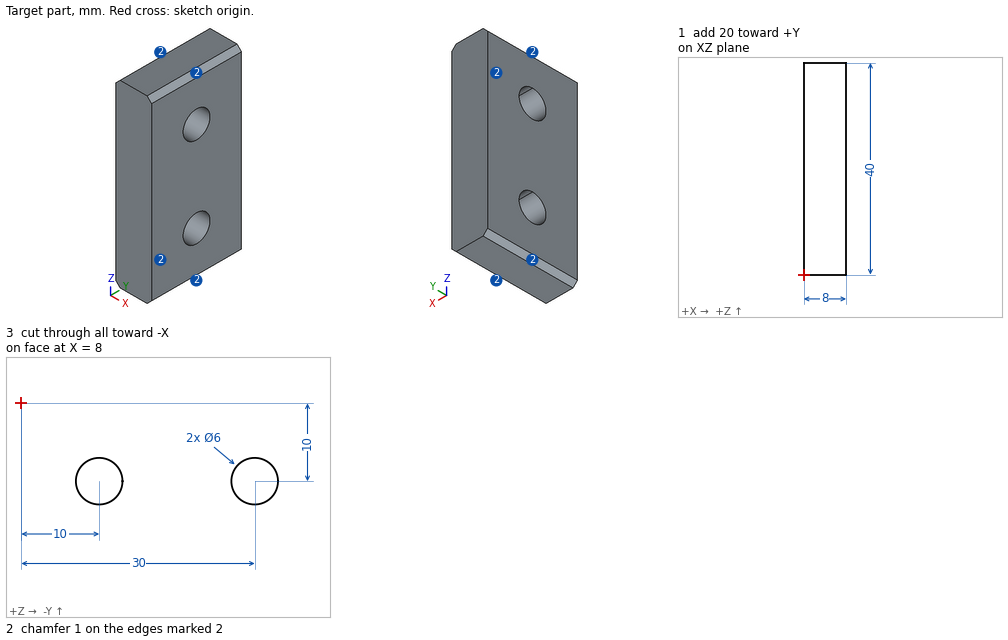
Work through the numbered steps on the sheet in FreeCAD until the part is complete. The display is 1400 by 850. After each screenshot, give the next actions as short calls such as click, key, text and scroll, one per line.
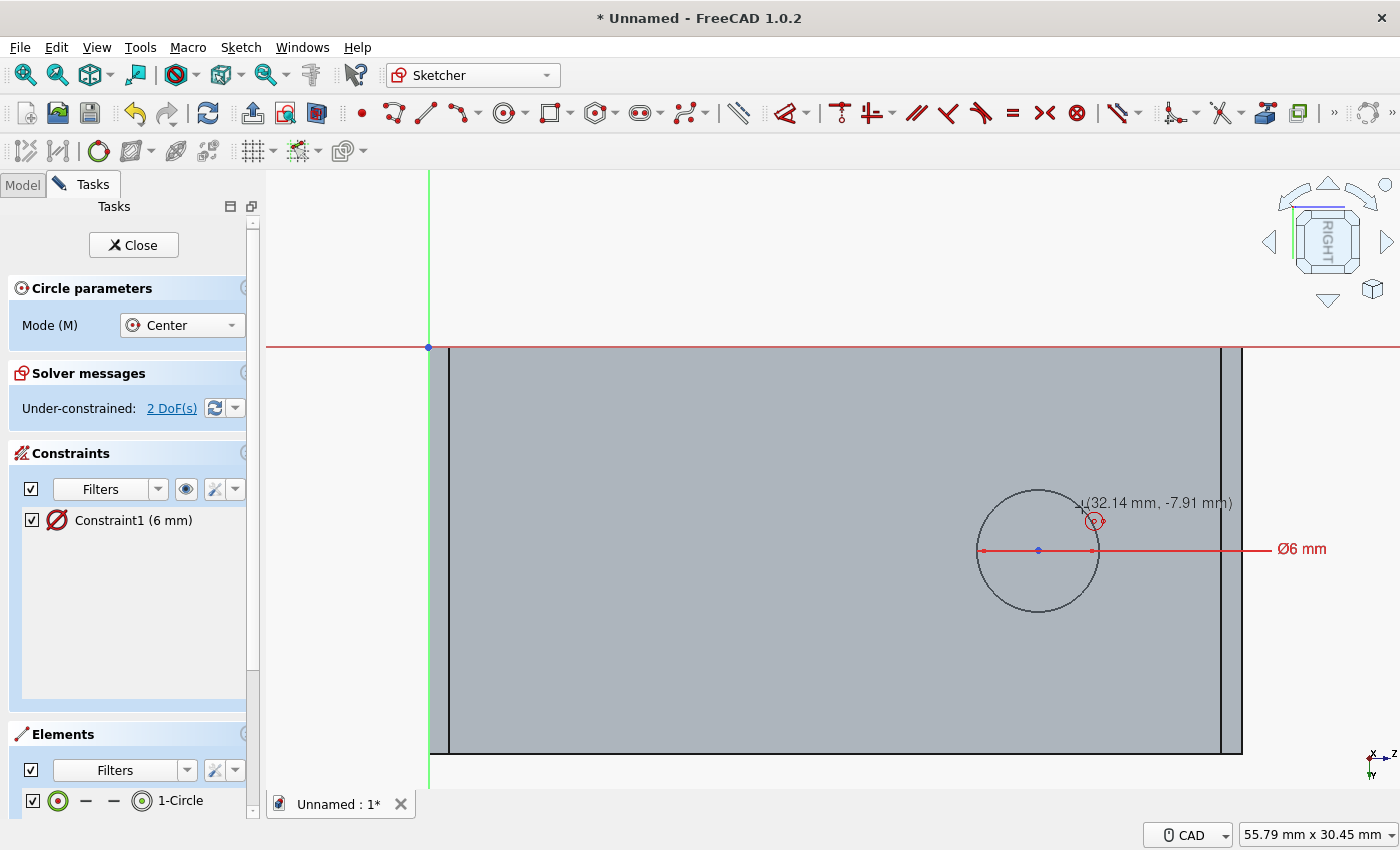
click(632, 550)
move(675, 507)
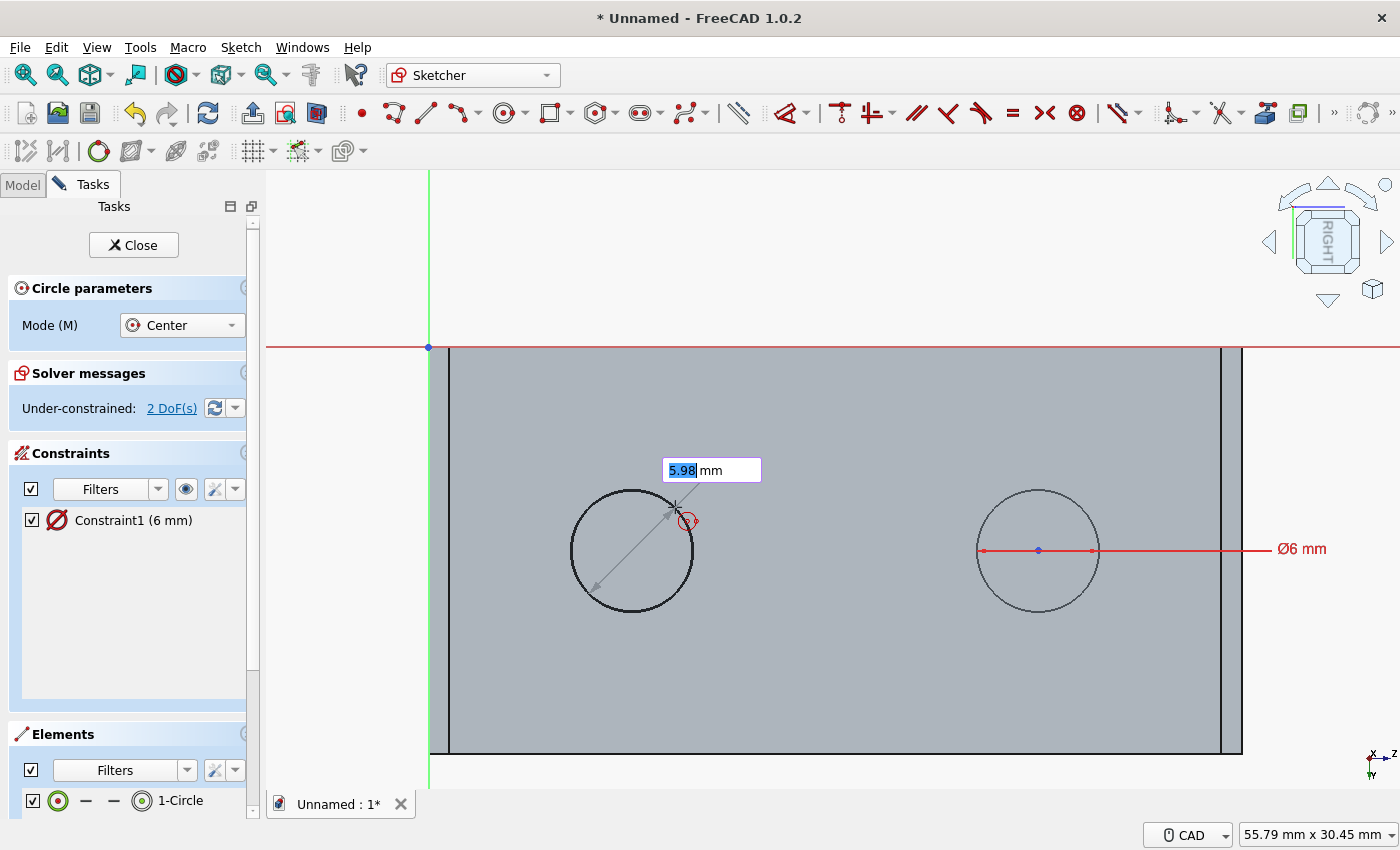
text(6)
key(Return)
key(Escape)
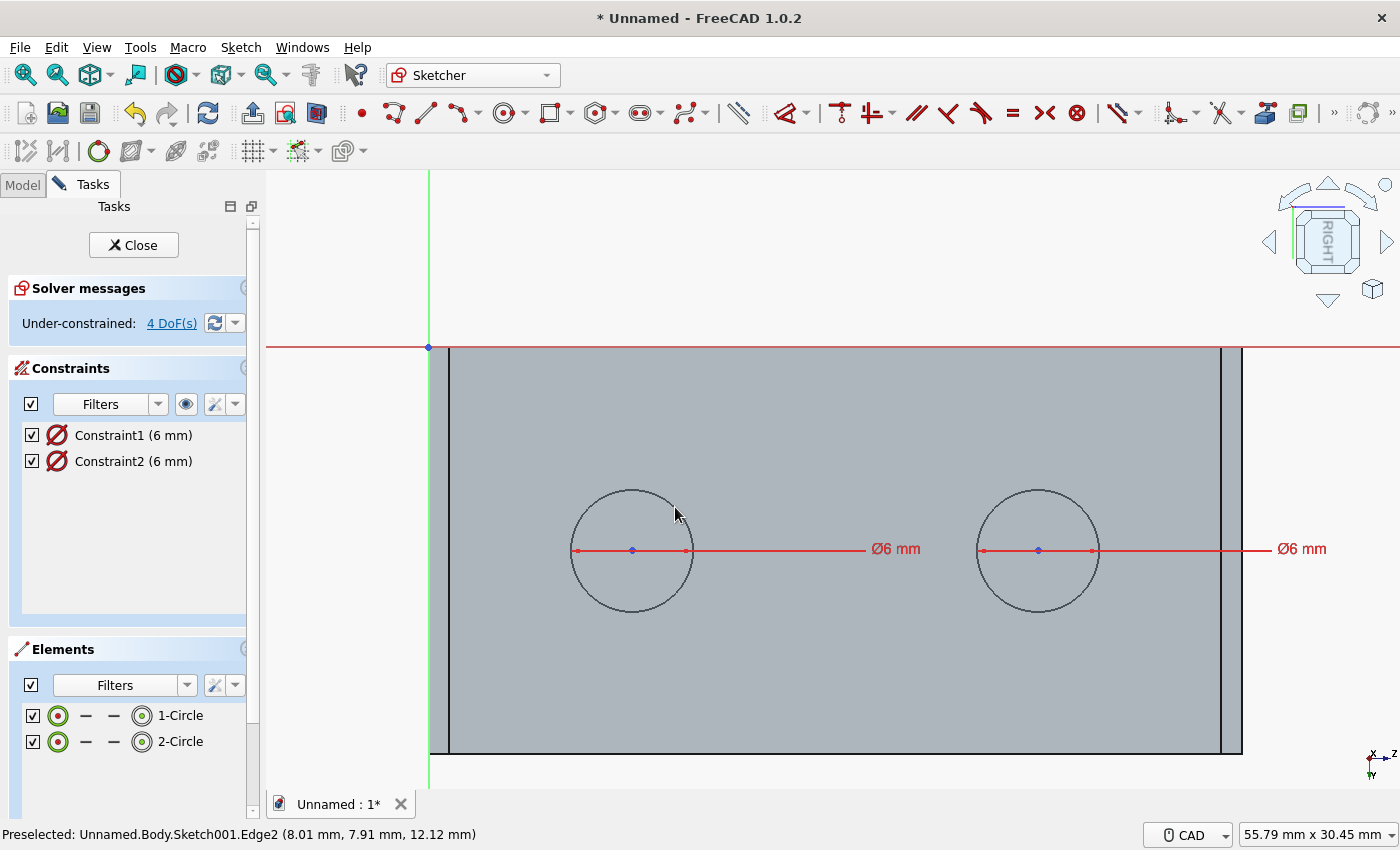
click(1038, 551)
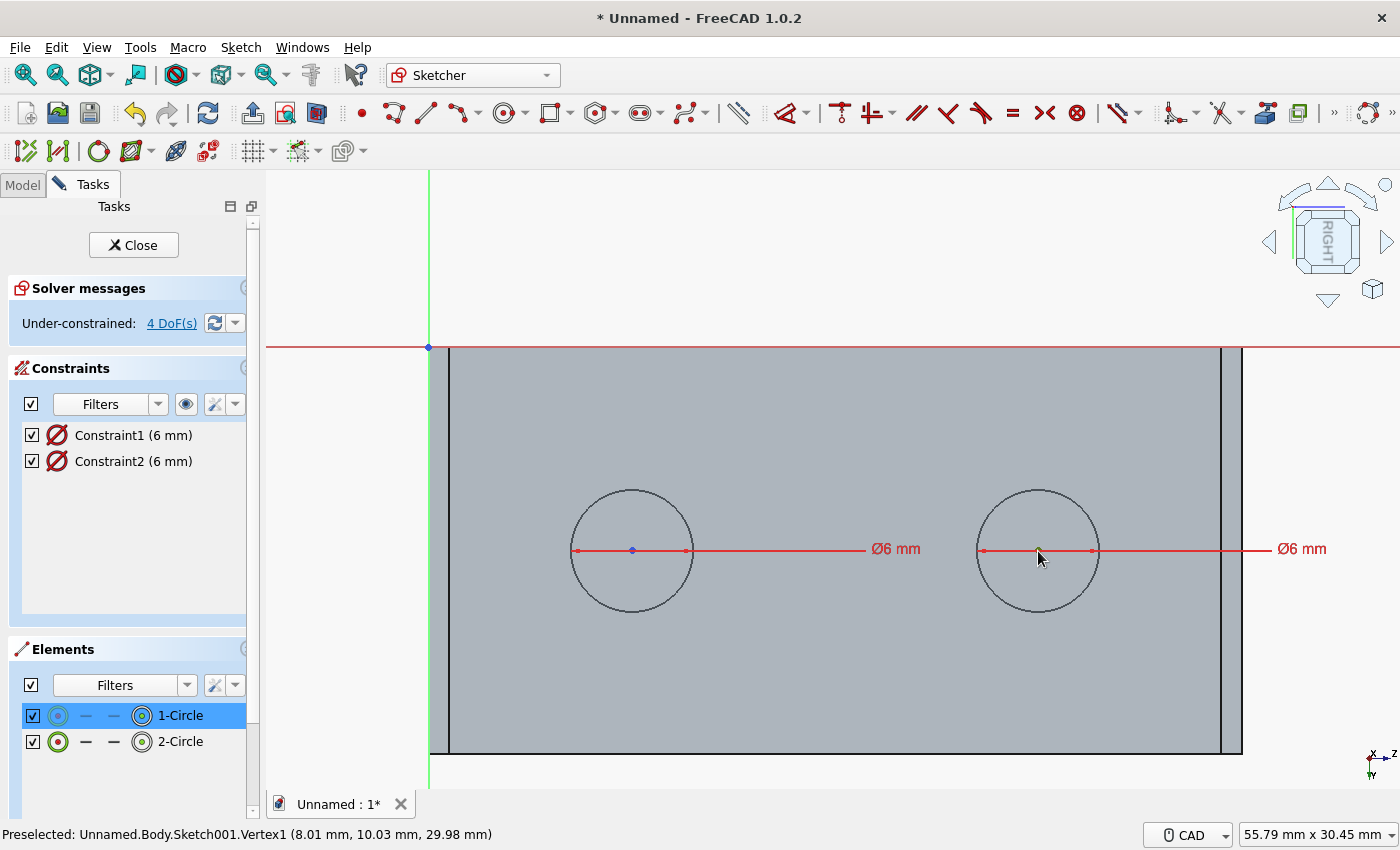
click(632, 551)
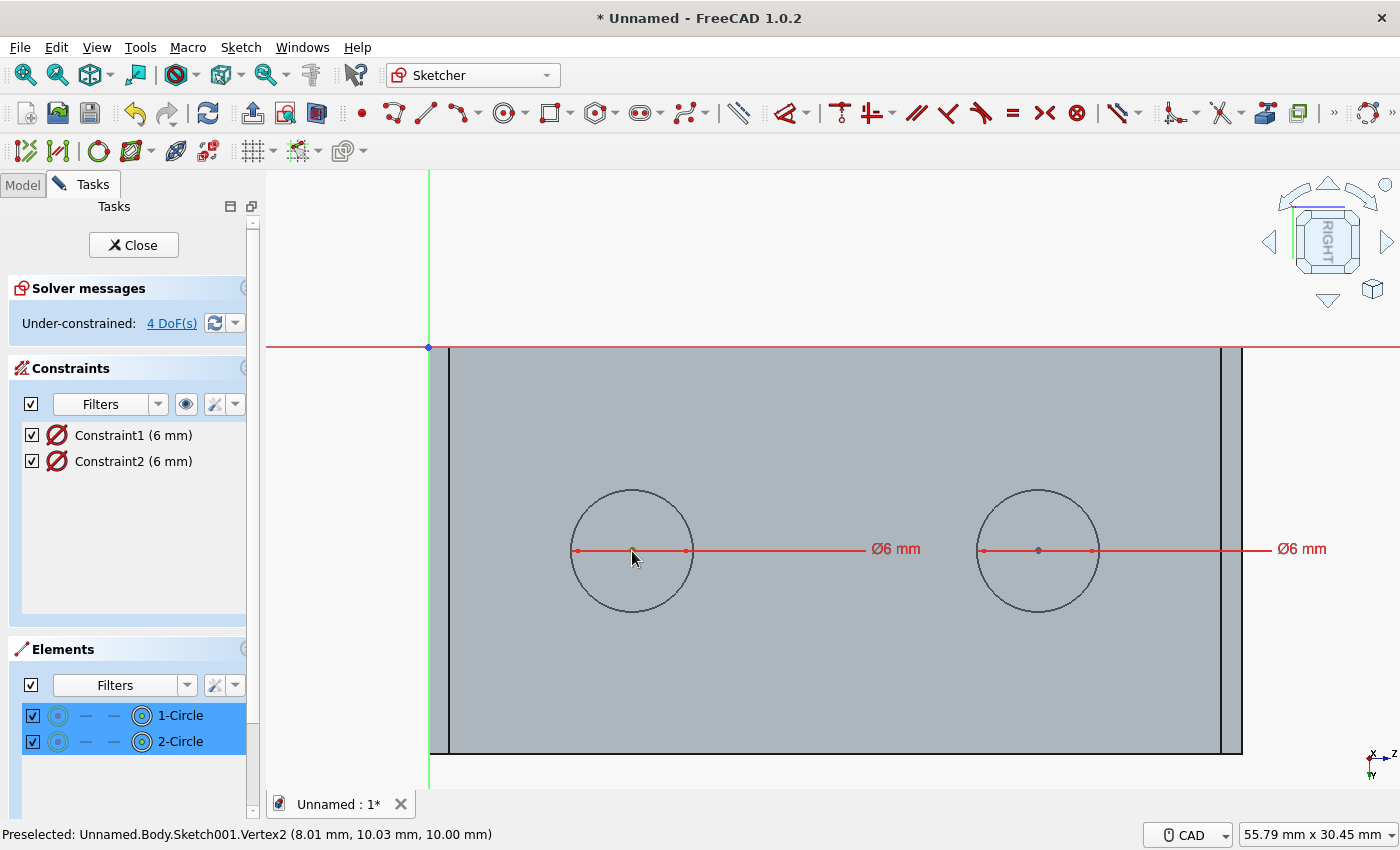
key(h)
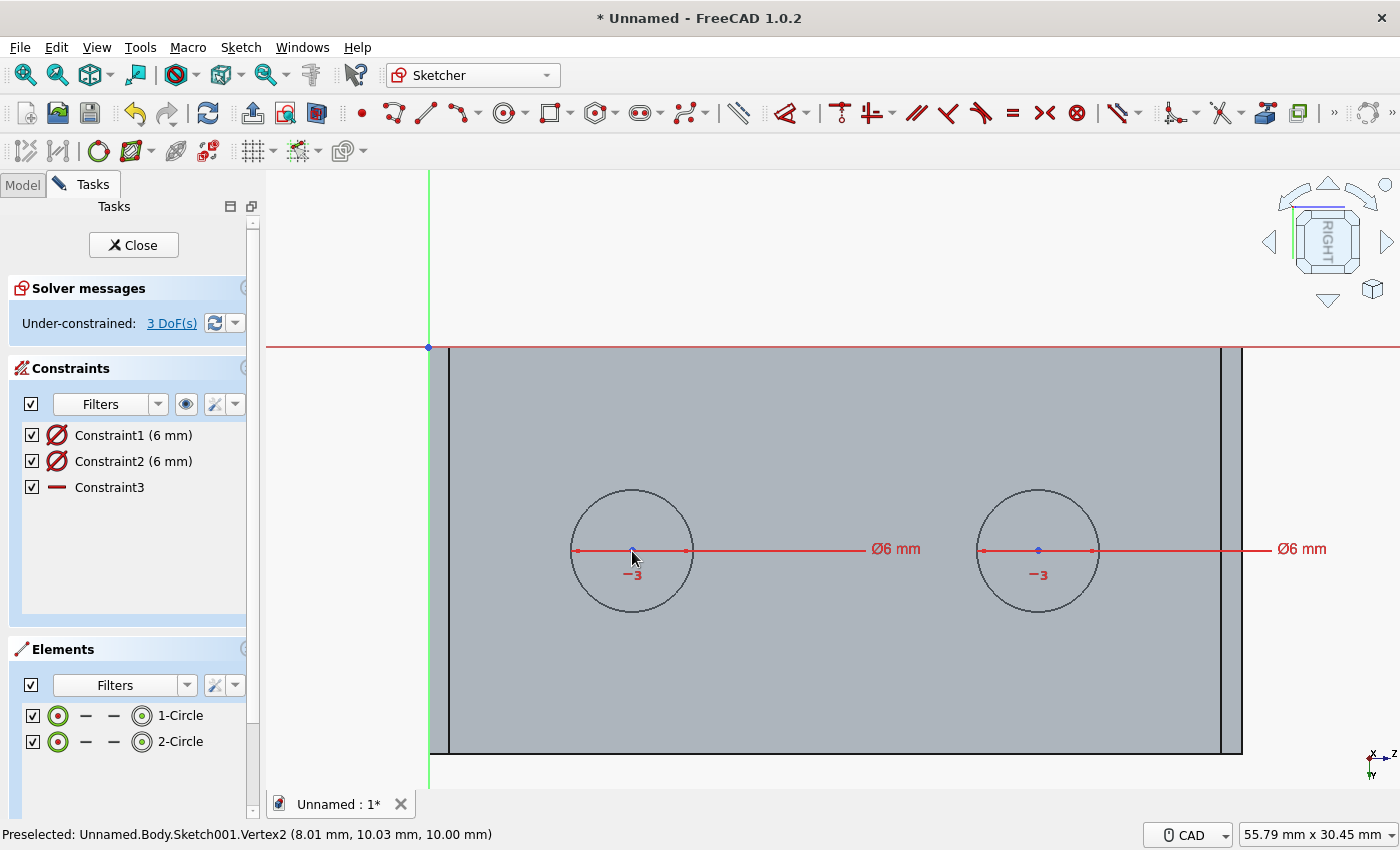
click(786, 114)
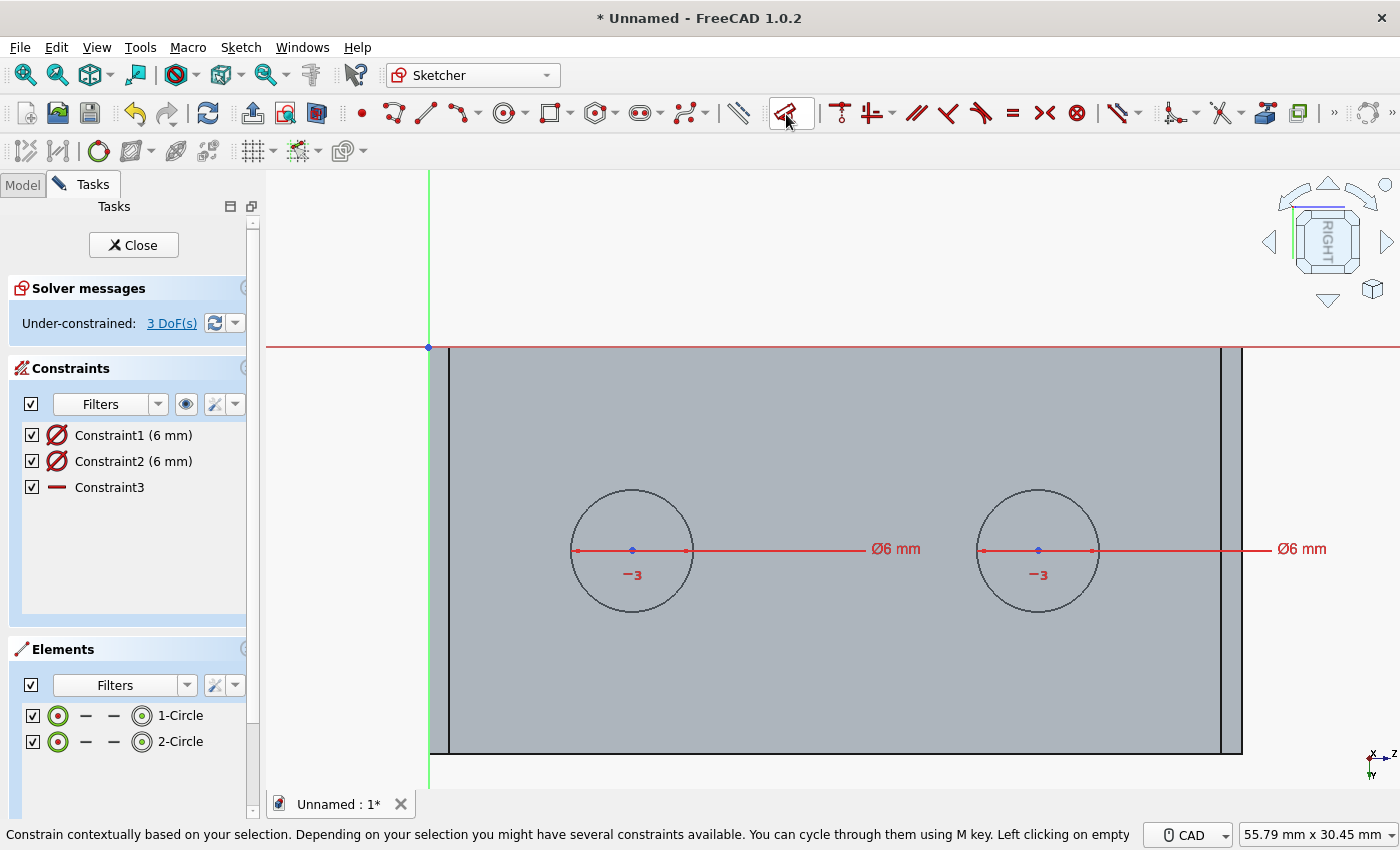
click(1038, 551)
click(733, 313)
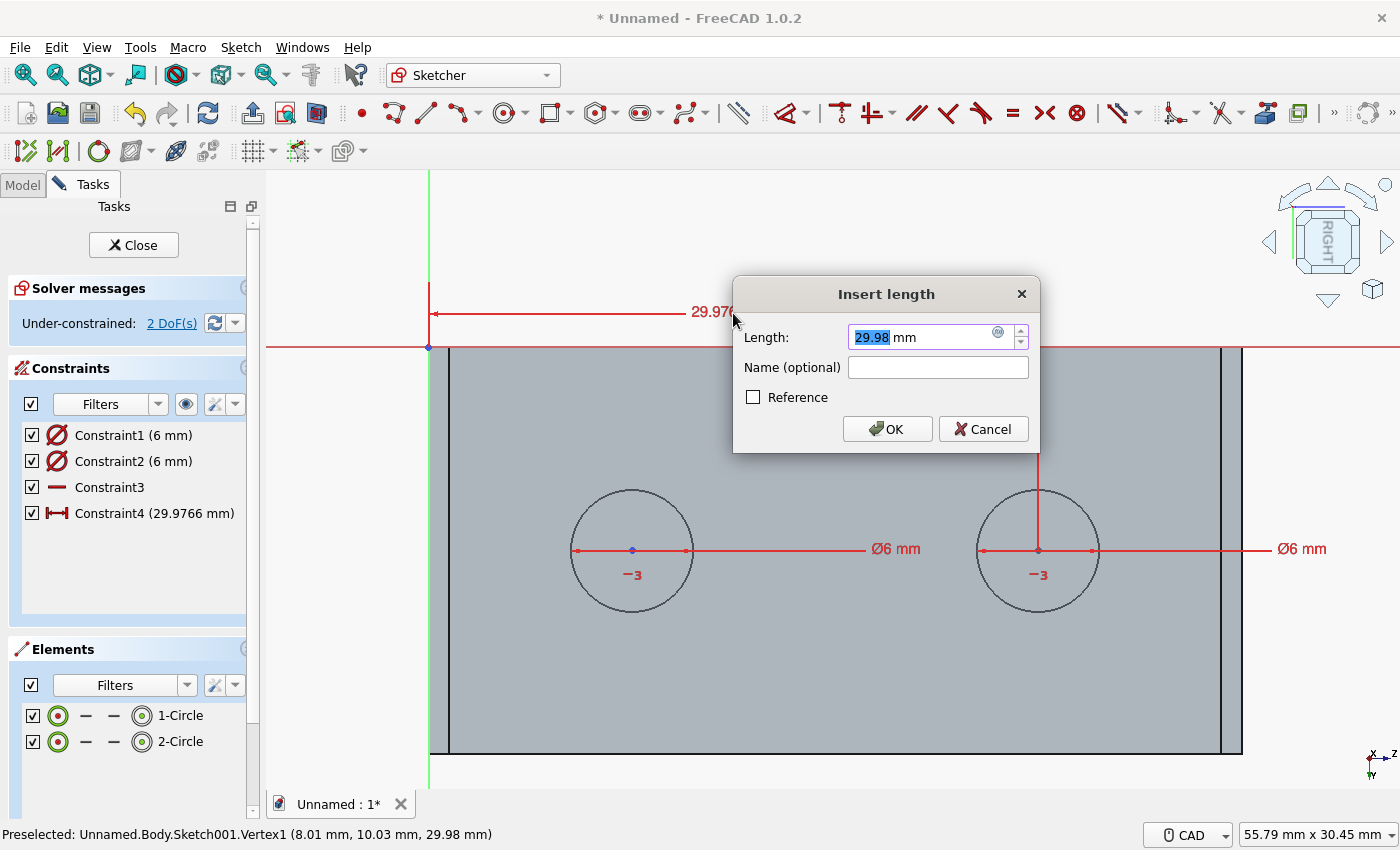
text(30)
key(Return)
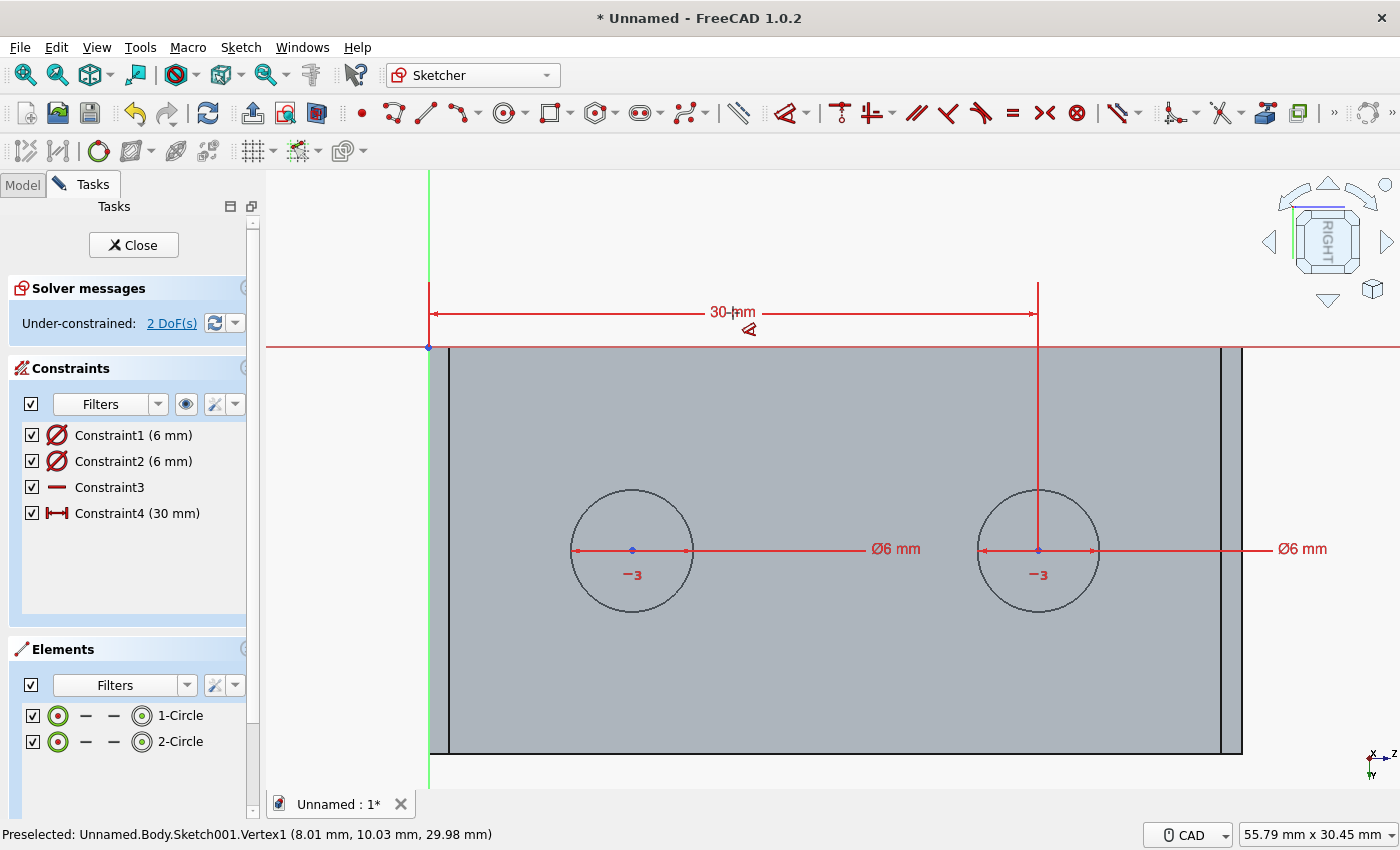
click(1038, 551)
click(395, 449)